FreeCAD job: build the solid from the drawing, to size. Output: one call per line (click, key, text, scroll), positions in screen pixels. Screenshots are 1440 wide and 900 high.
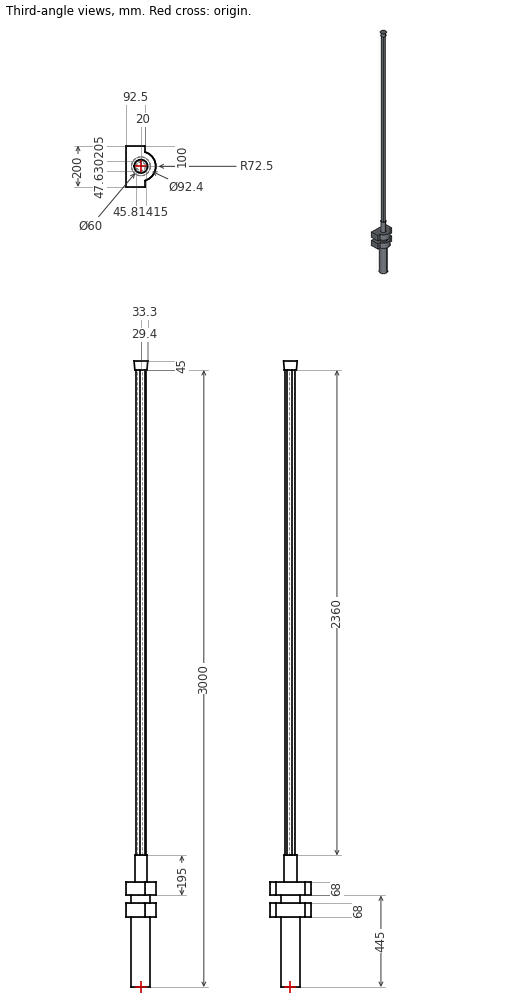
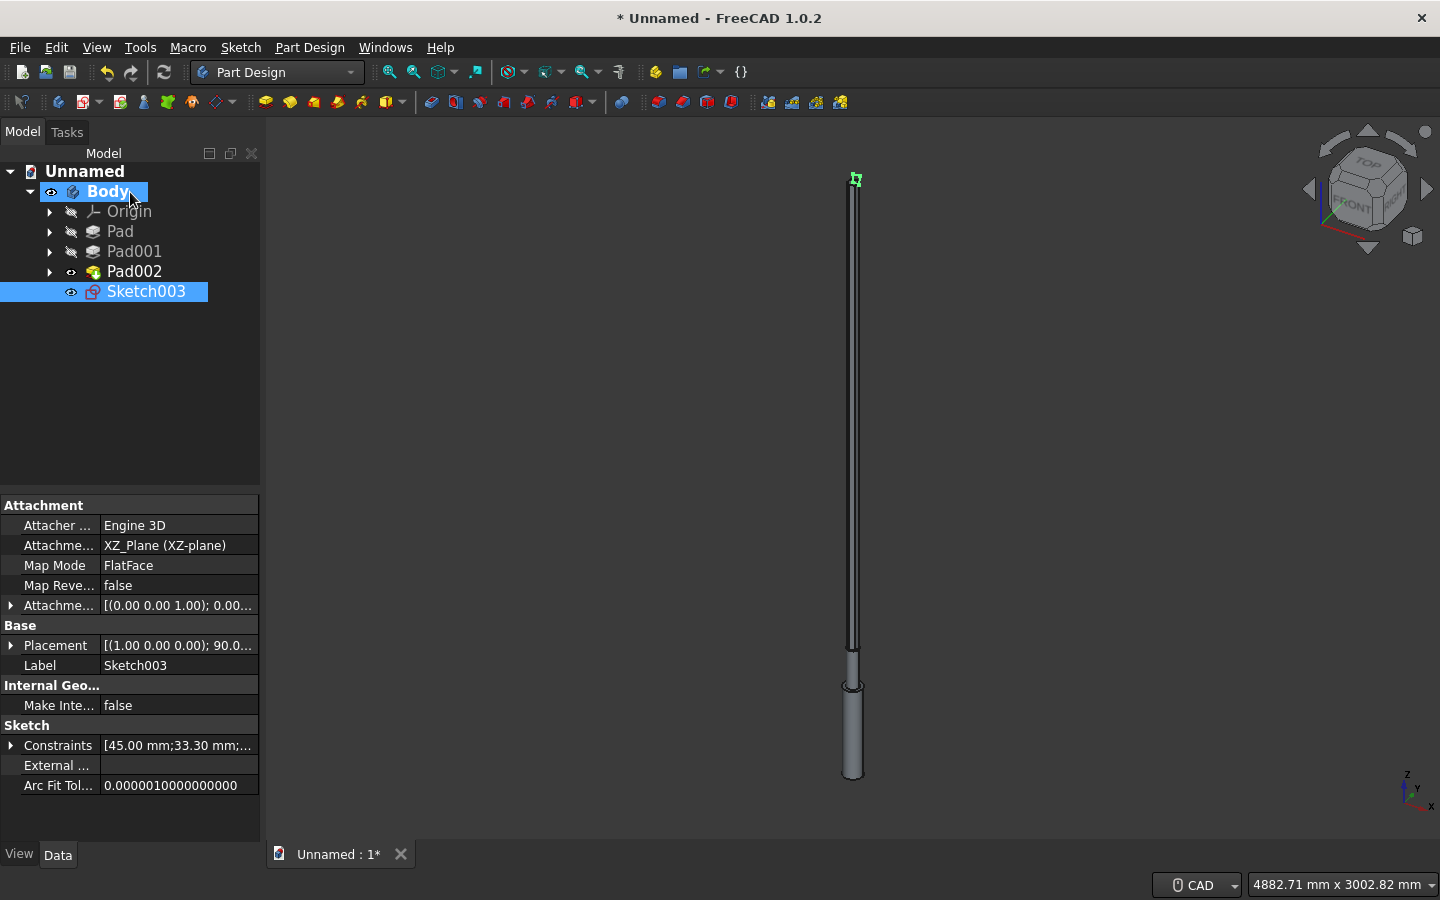
click(290, 102)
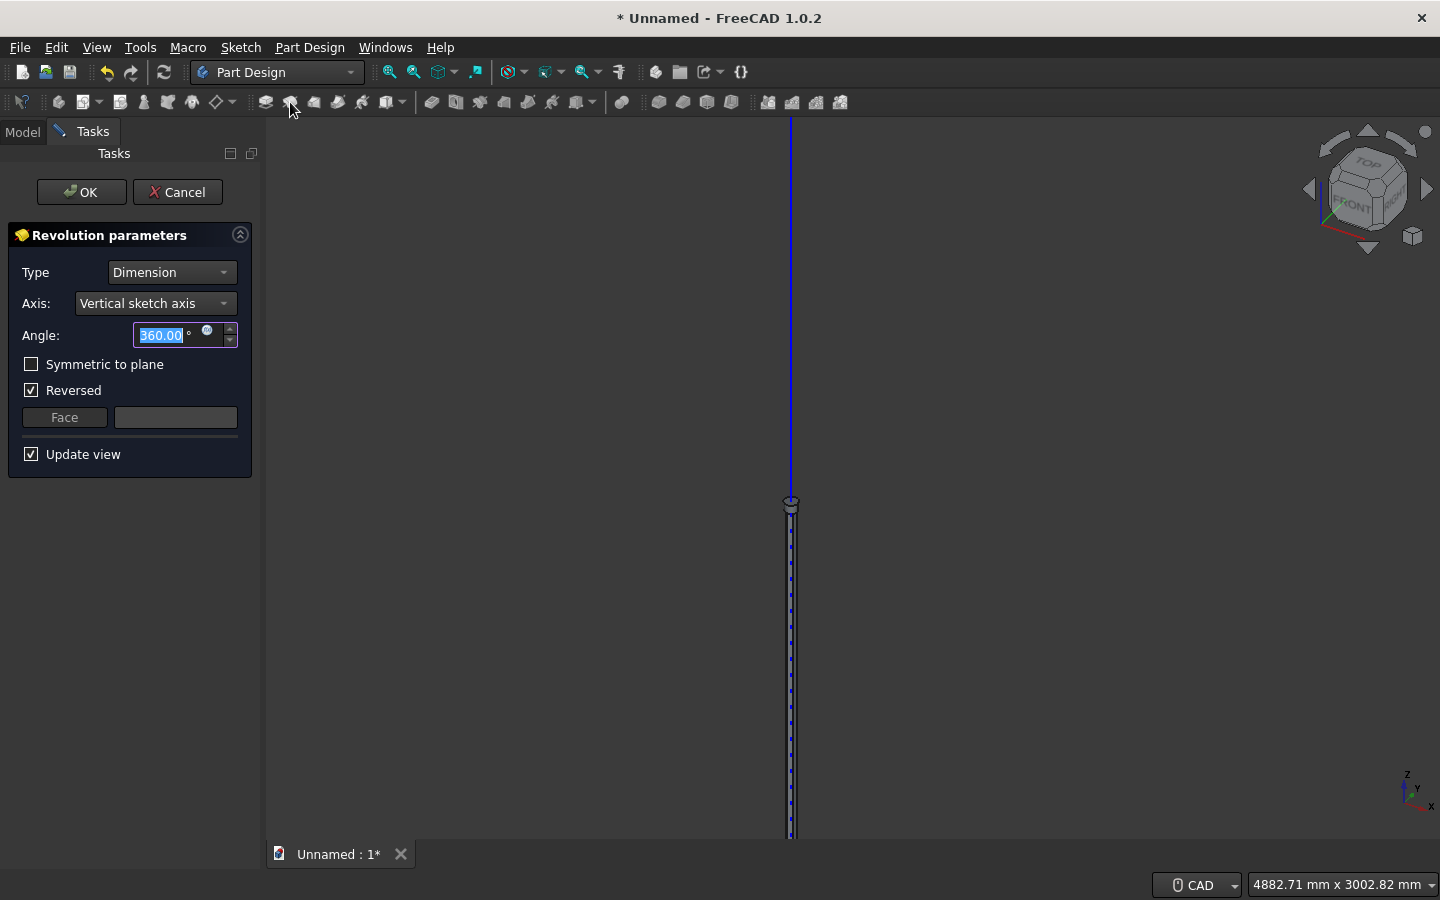
click(82, 192)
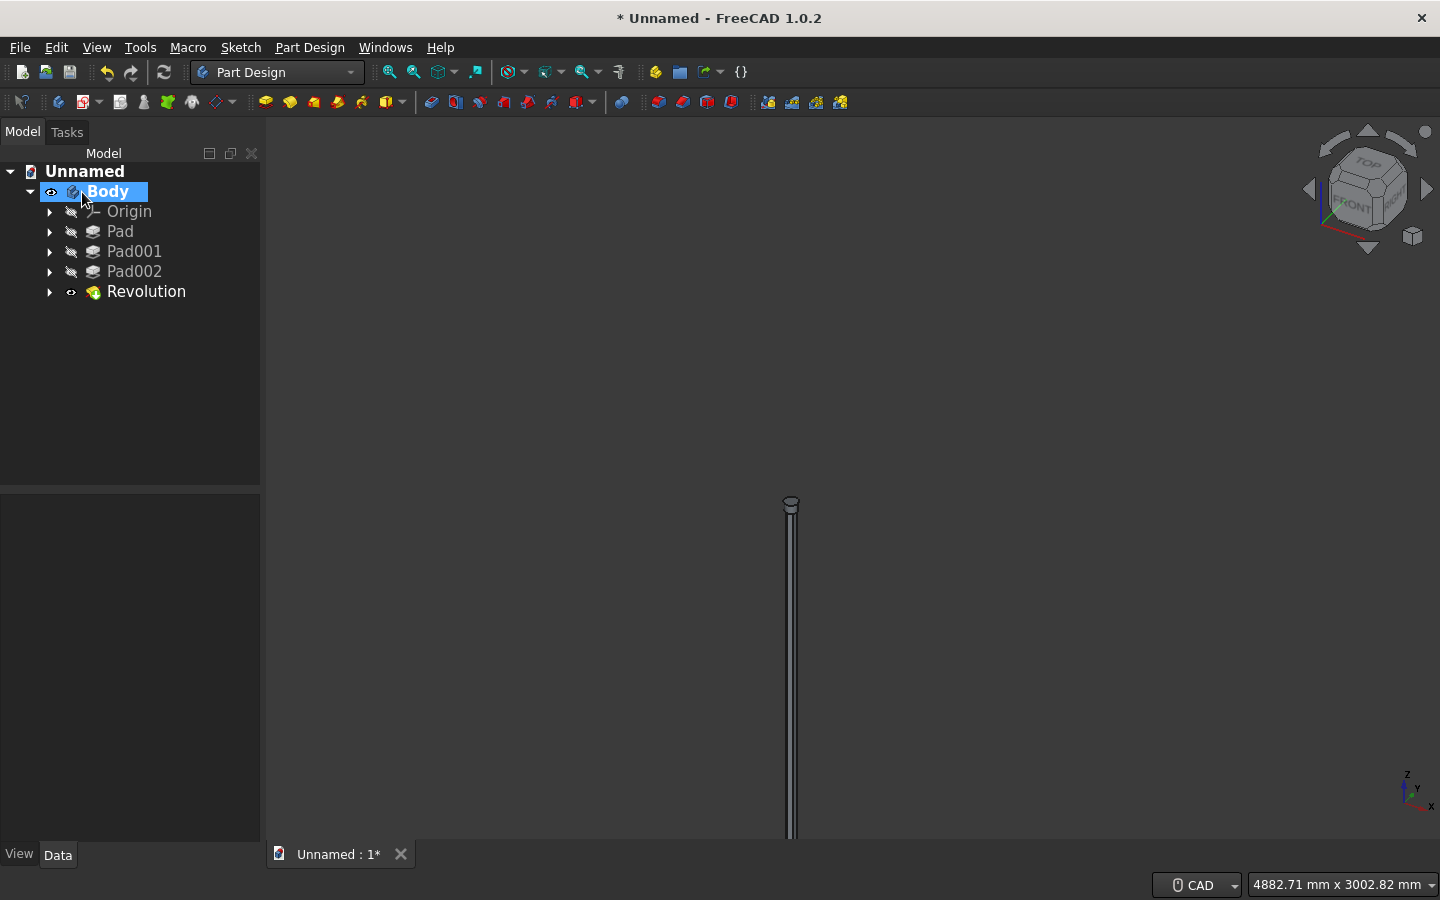
click(390, 72)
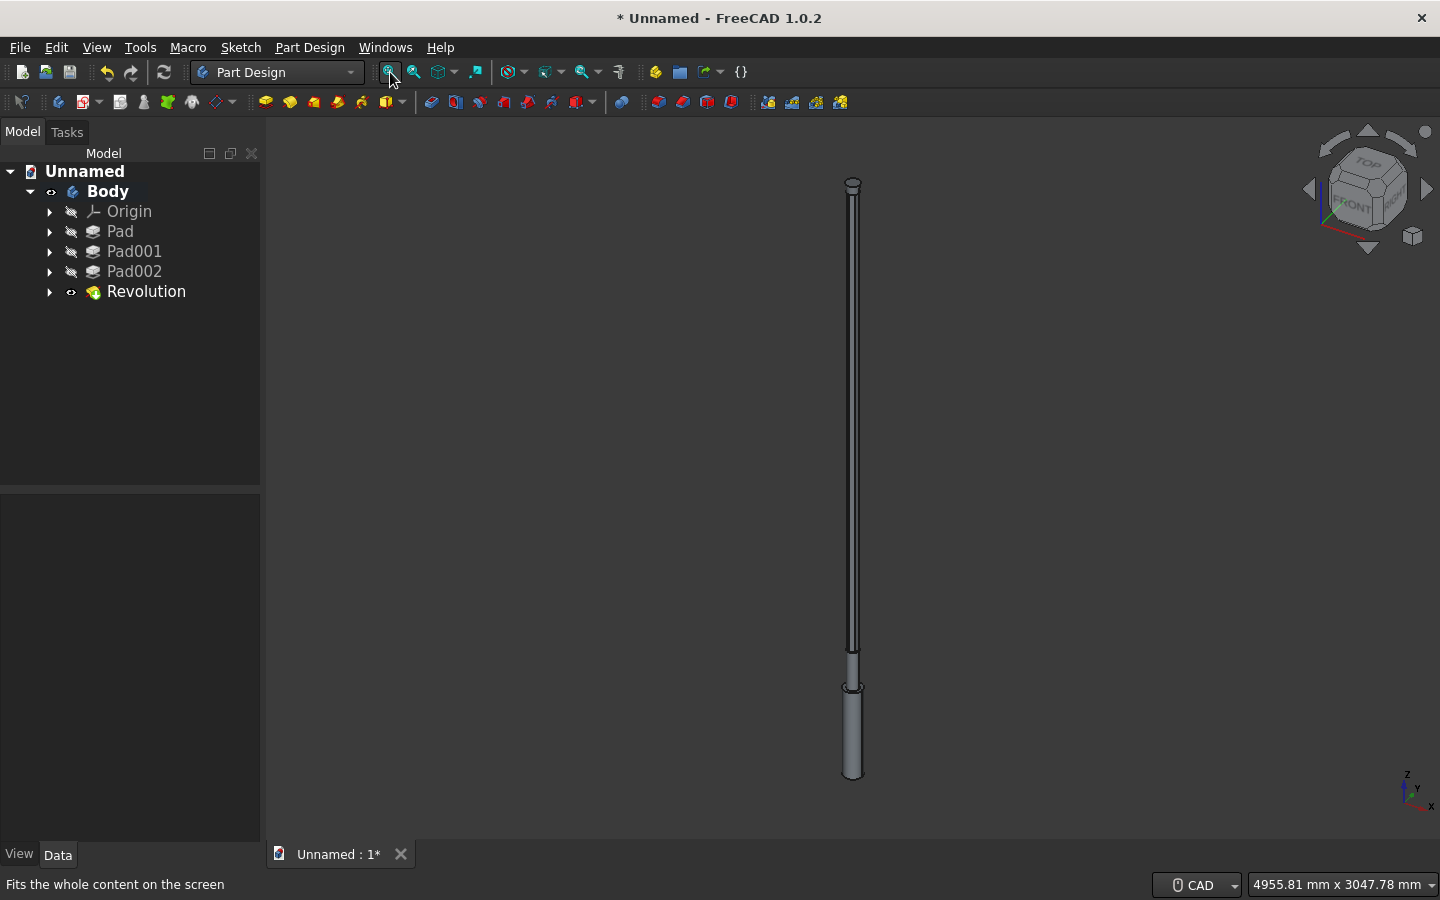
scroll(862, 685, up, 10)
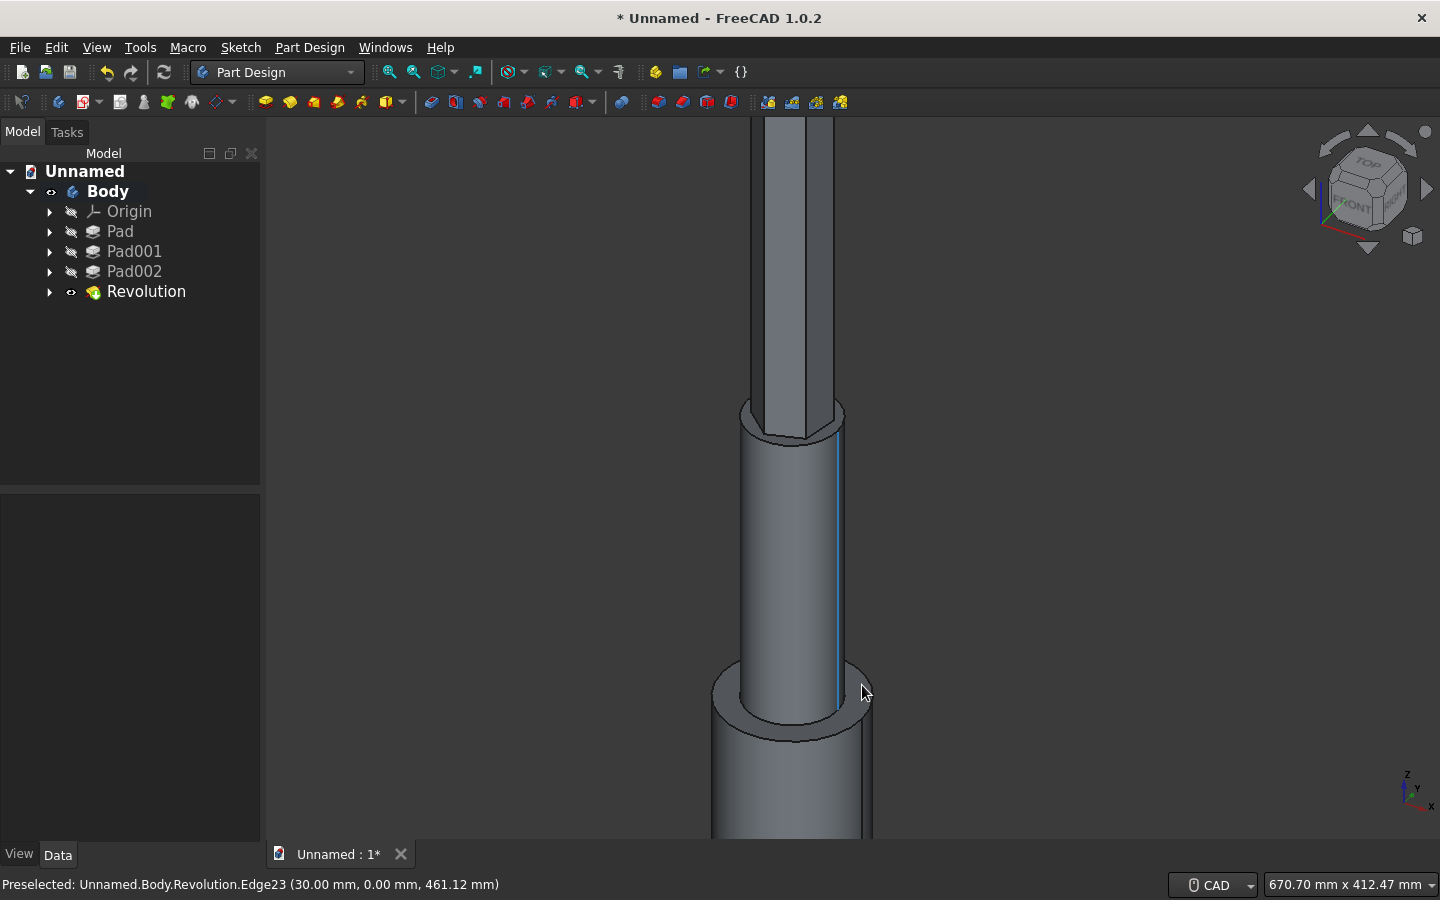
click(855, 685)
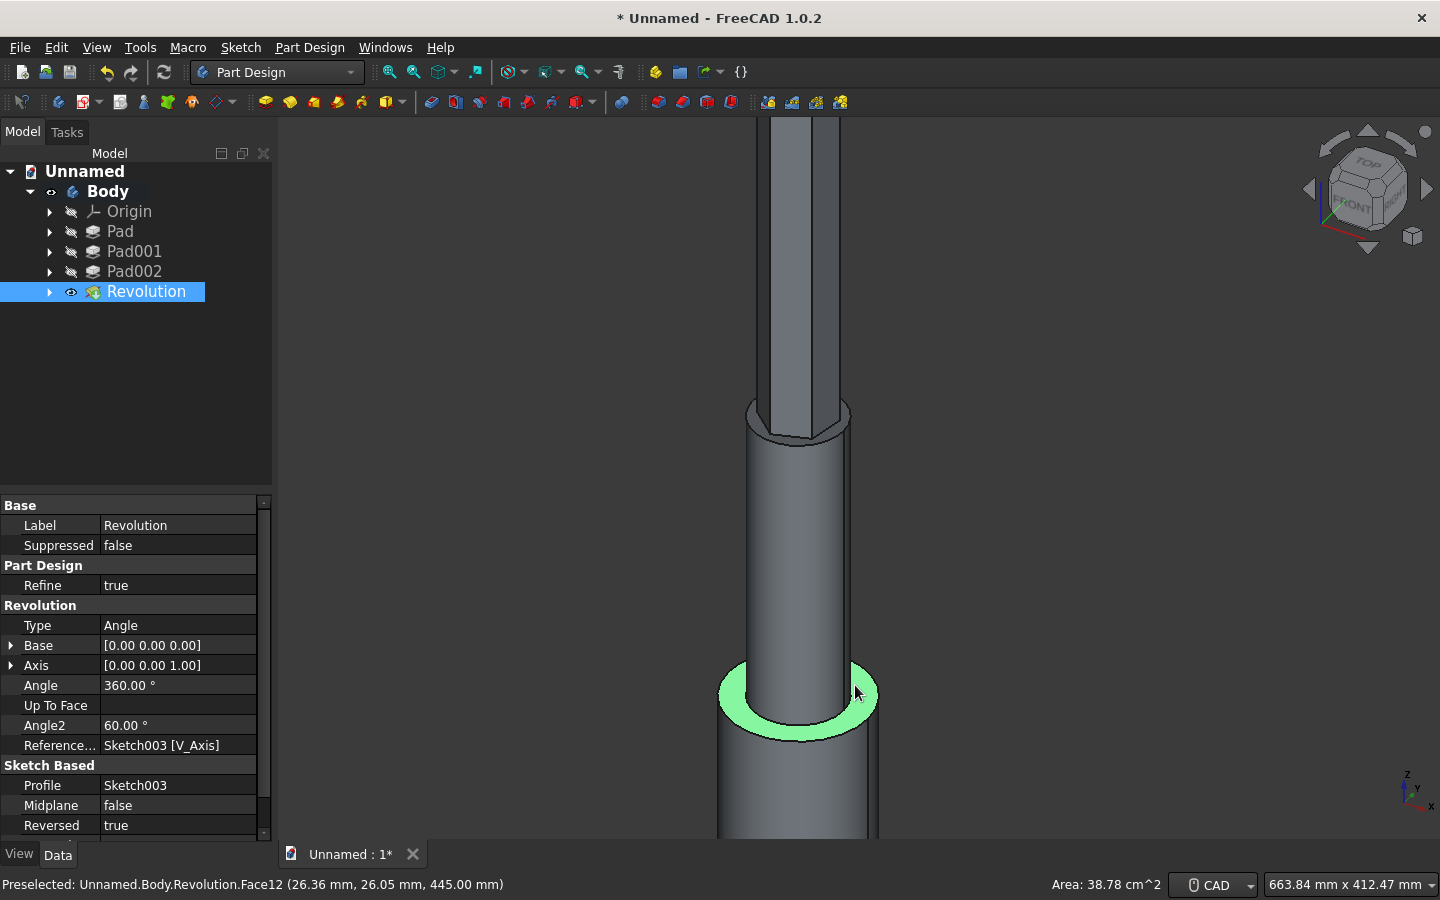
click(84, 102)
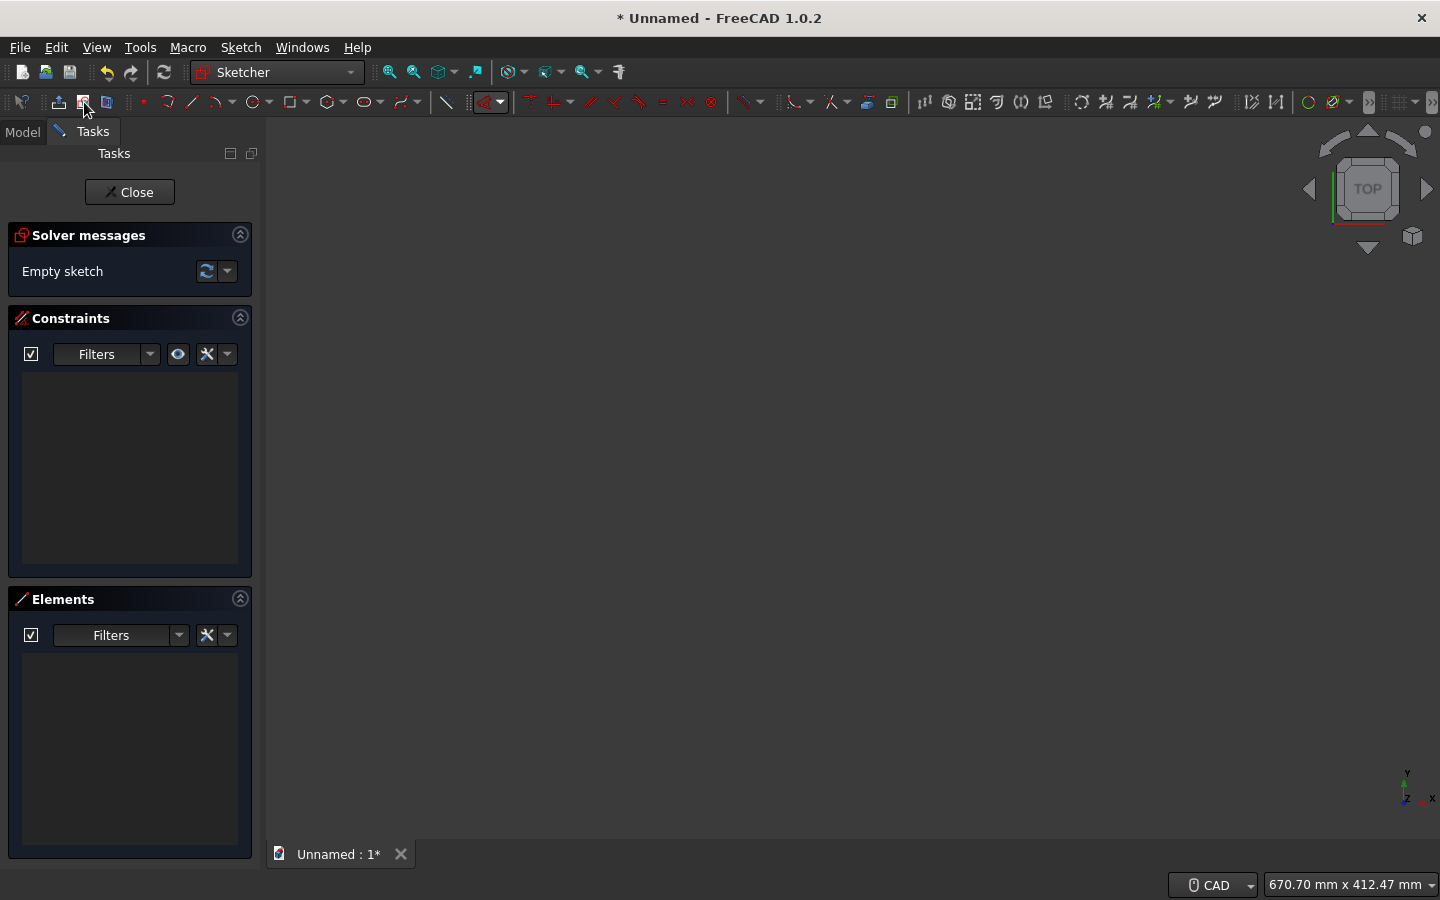
key(q)
key(s)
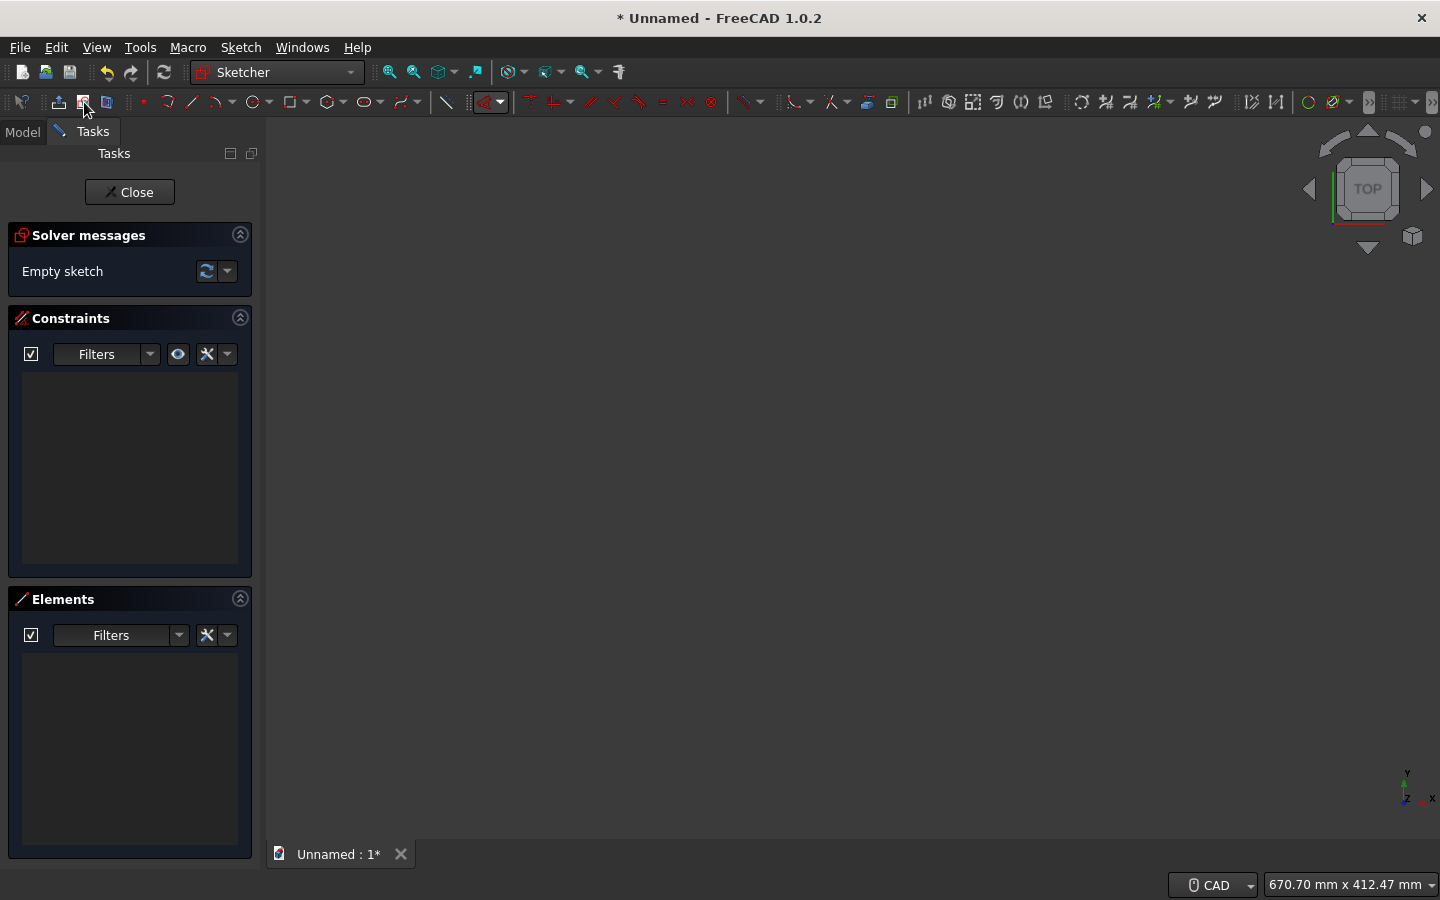
scroll(784, 478, down, 5)